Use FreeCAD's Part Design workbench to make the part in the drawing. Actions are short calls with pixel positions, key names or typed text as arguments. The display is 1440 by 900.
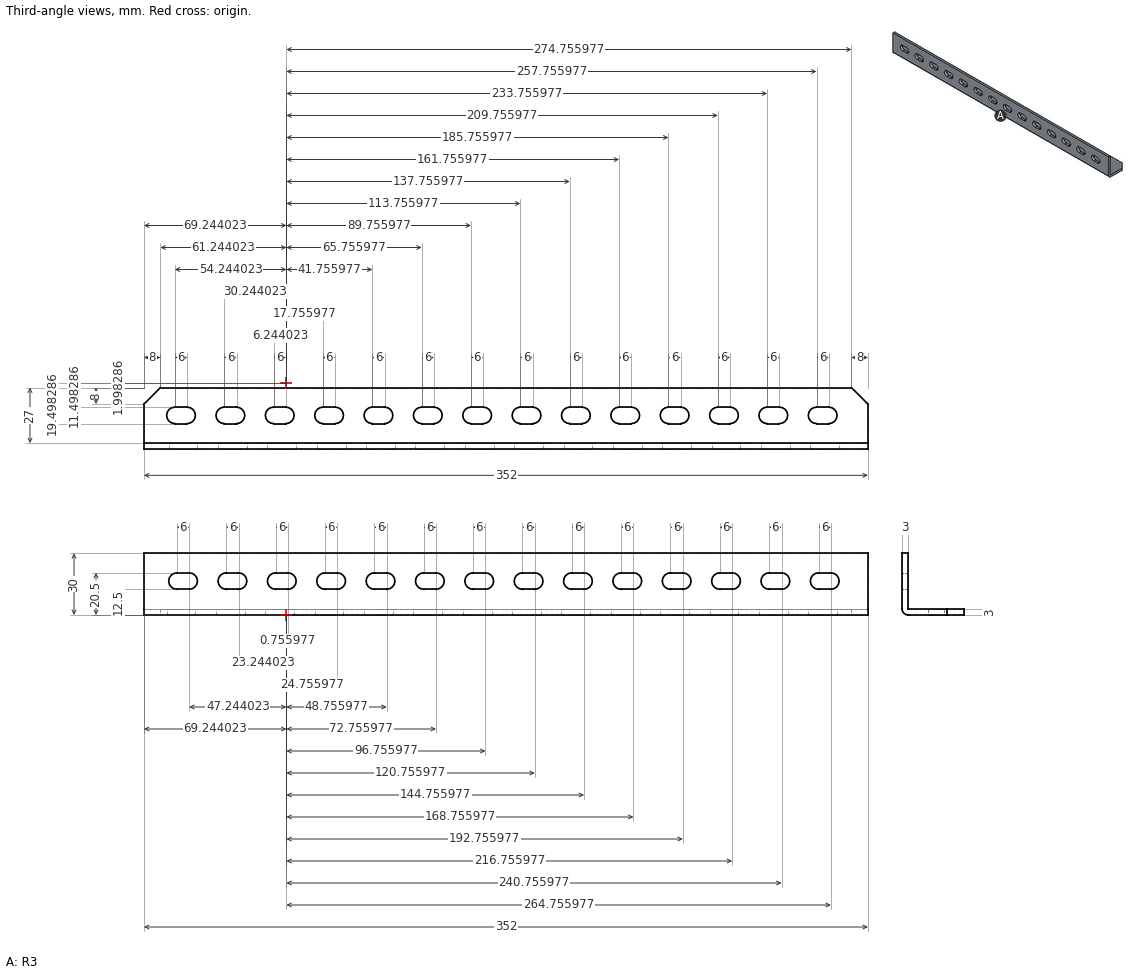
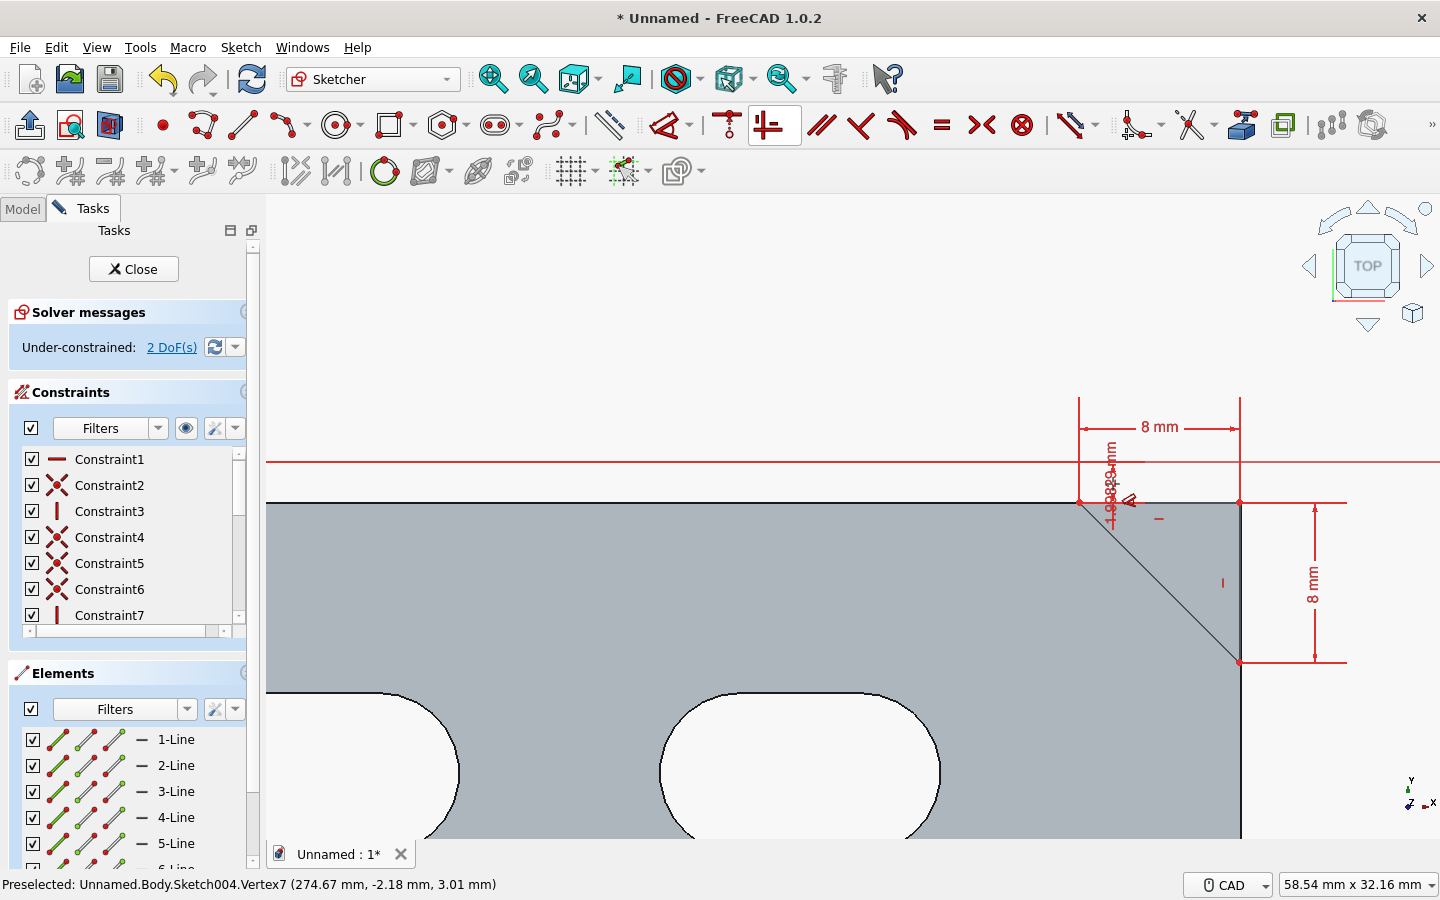
scroll(1091, 512, down, 12)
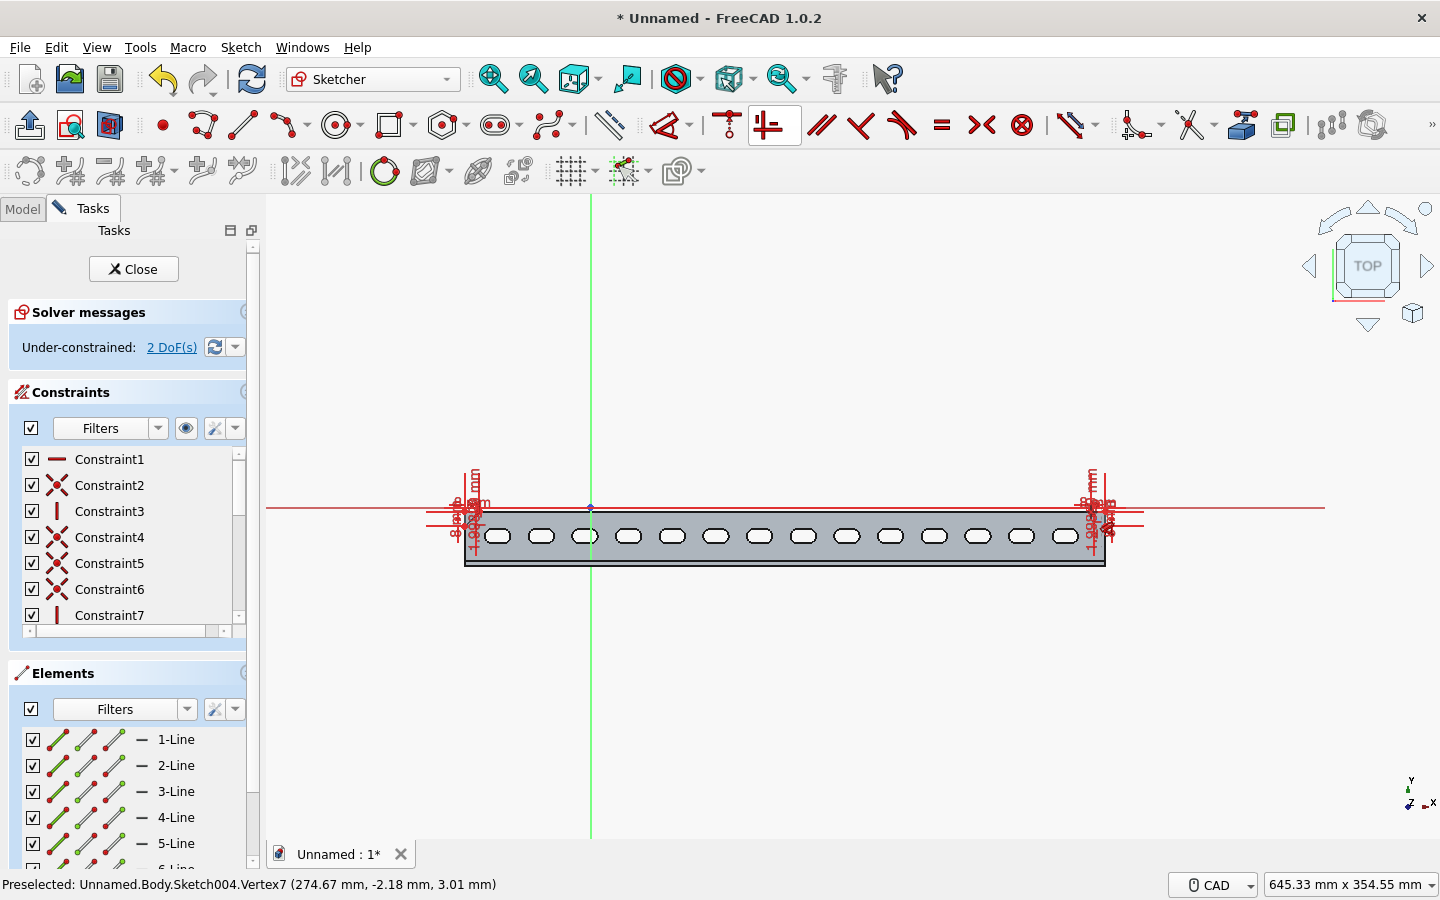
click(479, 512)
click(535, 474)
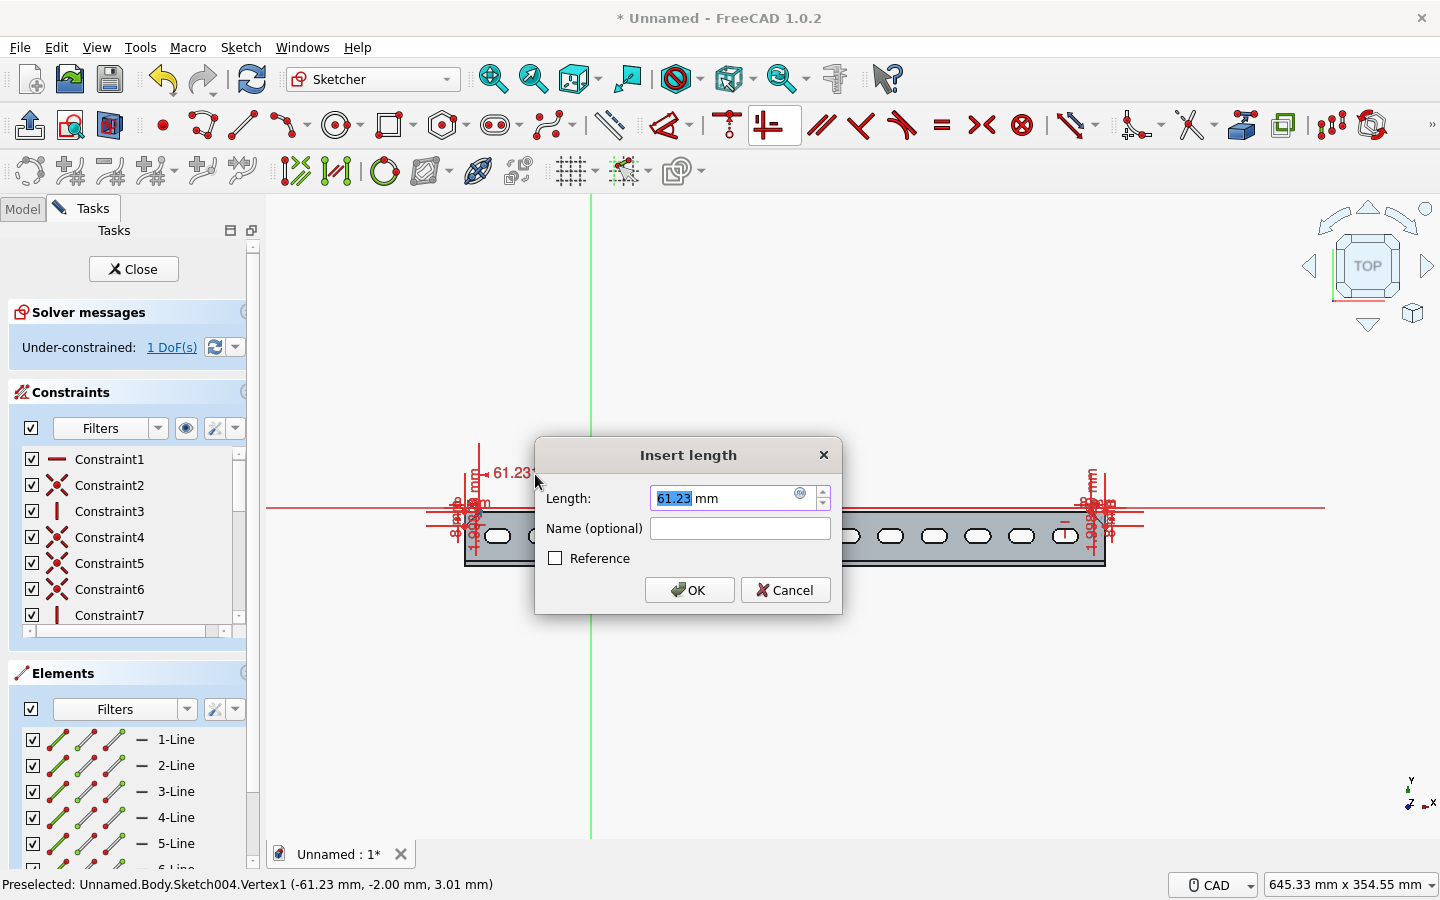
text(61.244023)
key(Return)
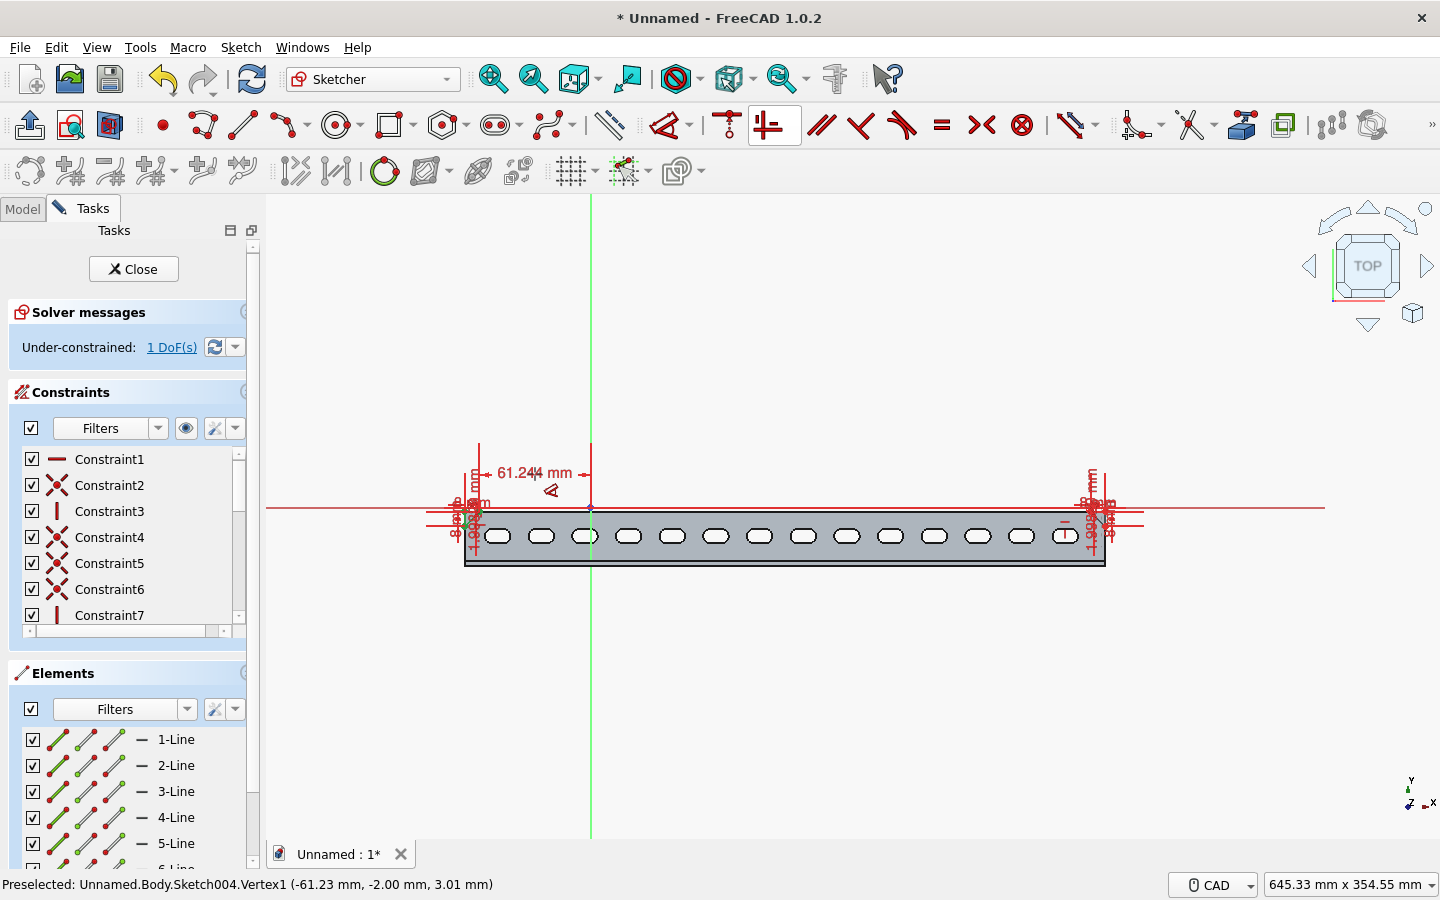
click(1091, 512)
click(841, 474)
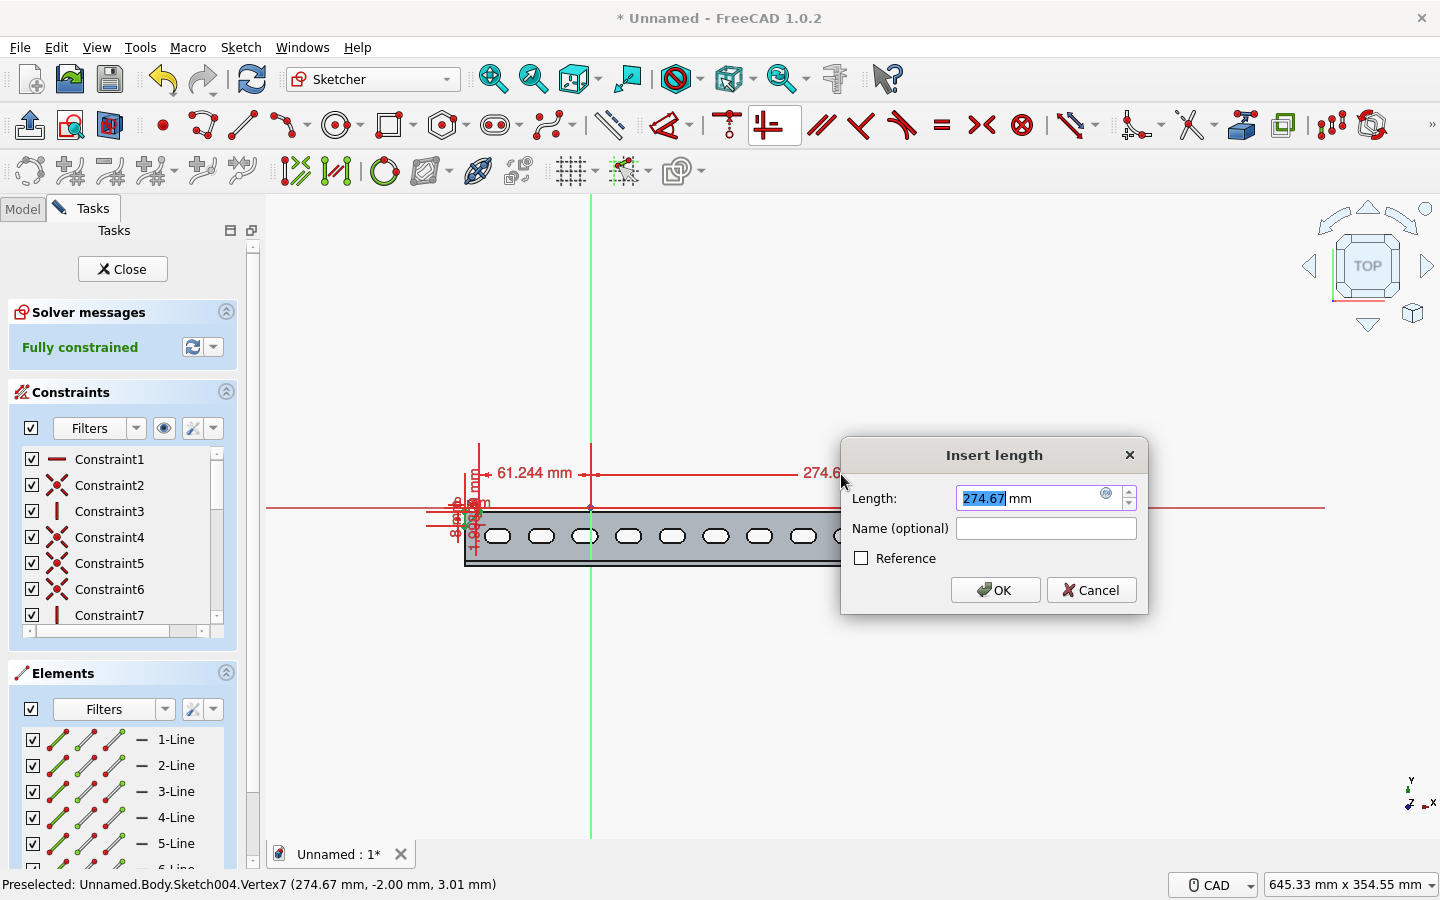
text(274.755977)
key(Return)
key(Escape)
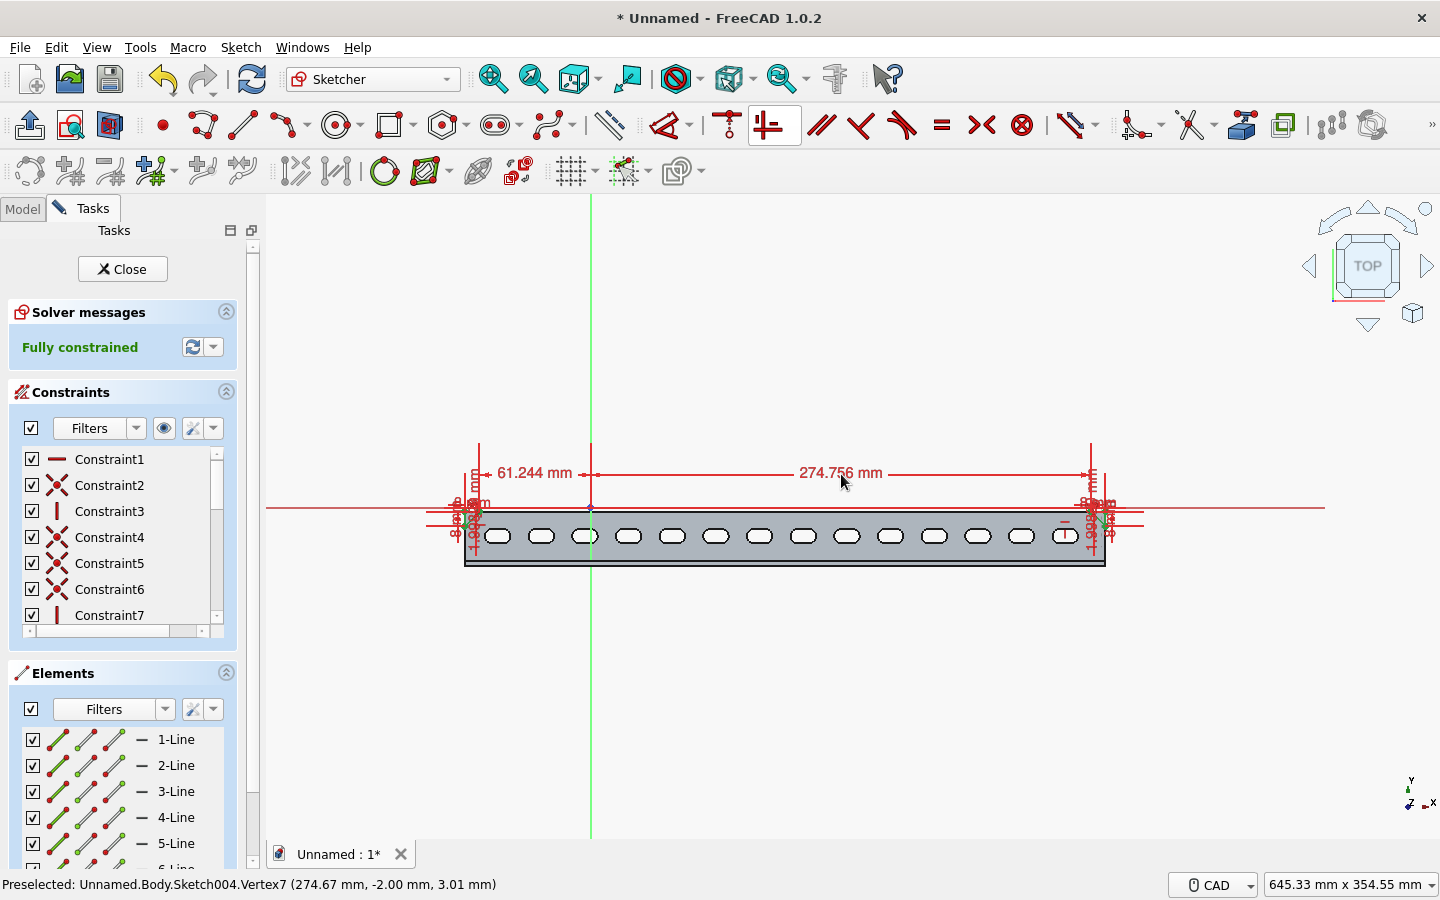
click(123, 269)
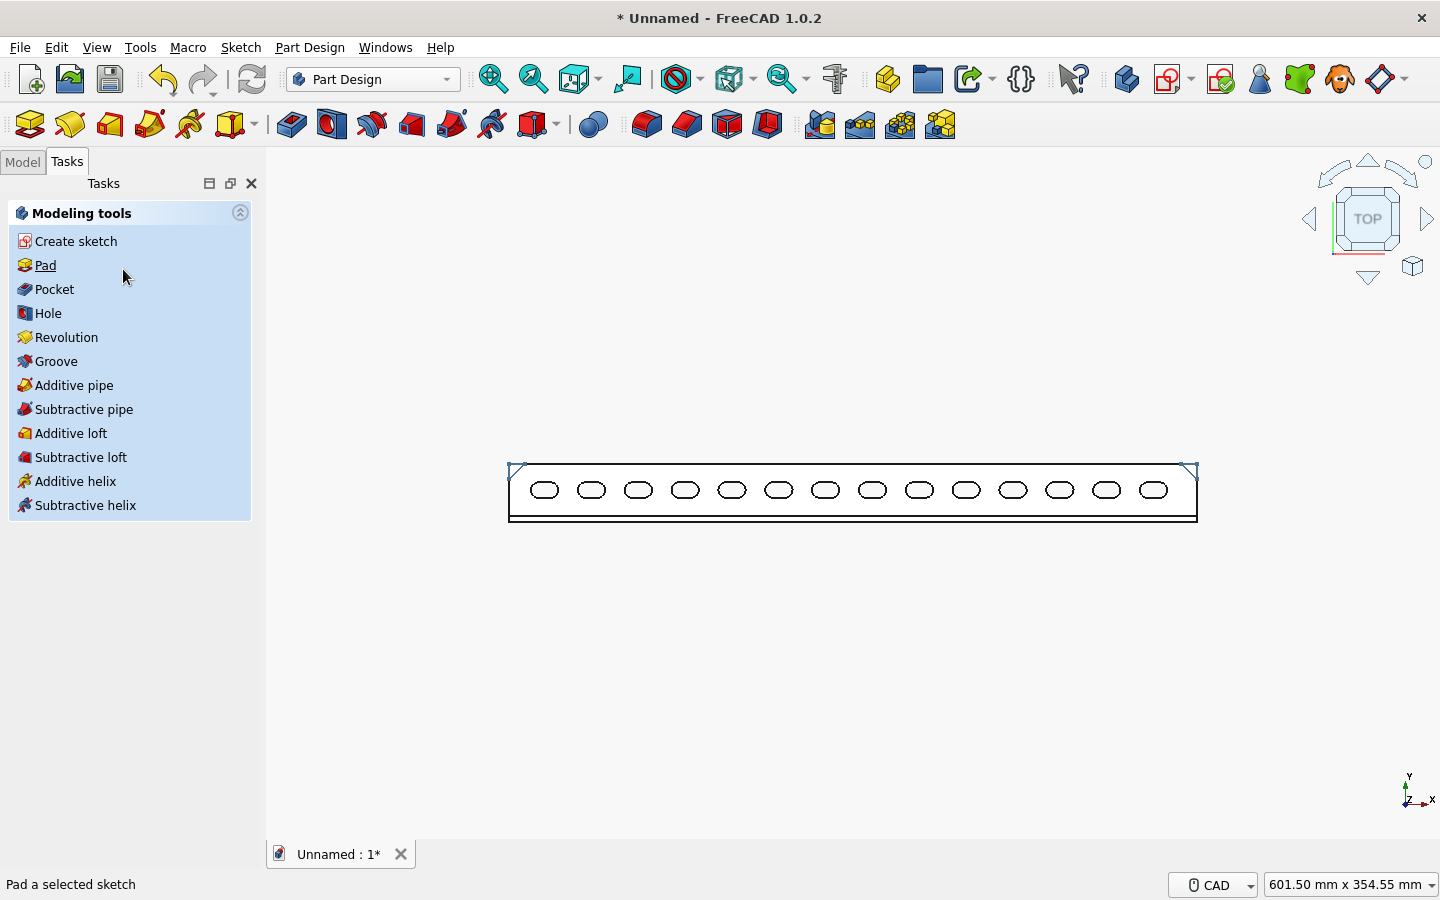
click(292, 124)